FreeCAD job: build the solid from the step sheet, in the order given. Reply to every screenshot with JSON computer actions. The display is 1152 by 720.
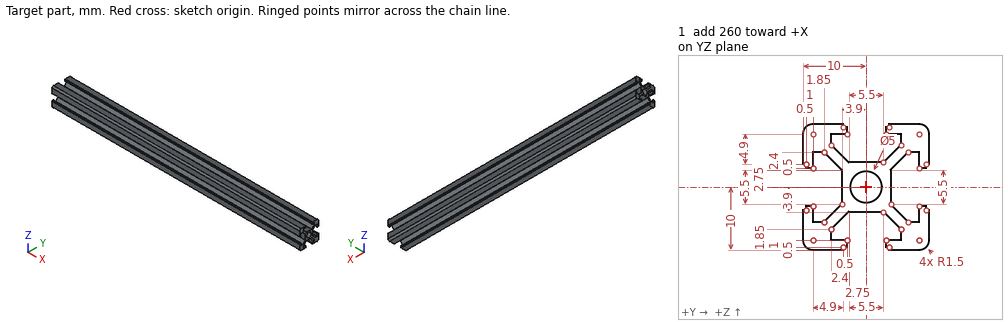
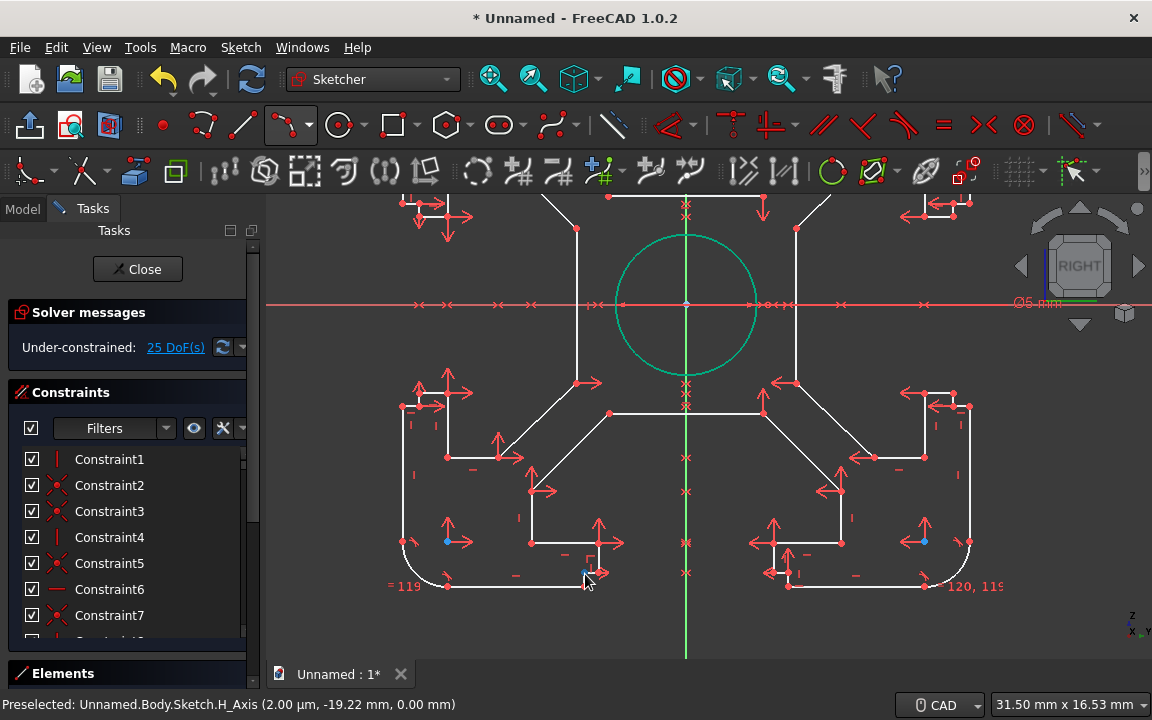
{"action": "left_click", "coordinate": [584, 573]}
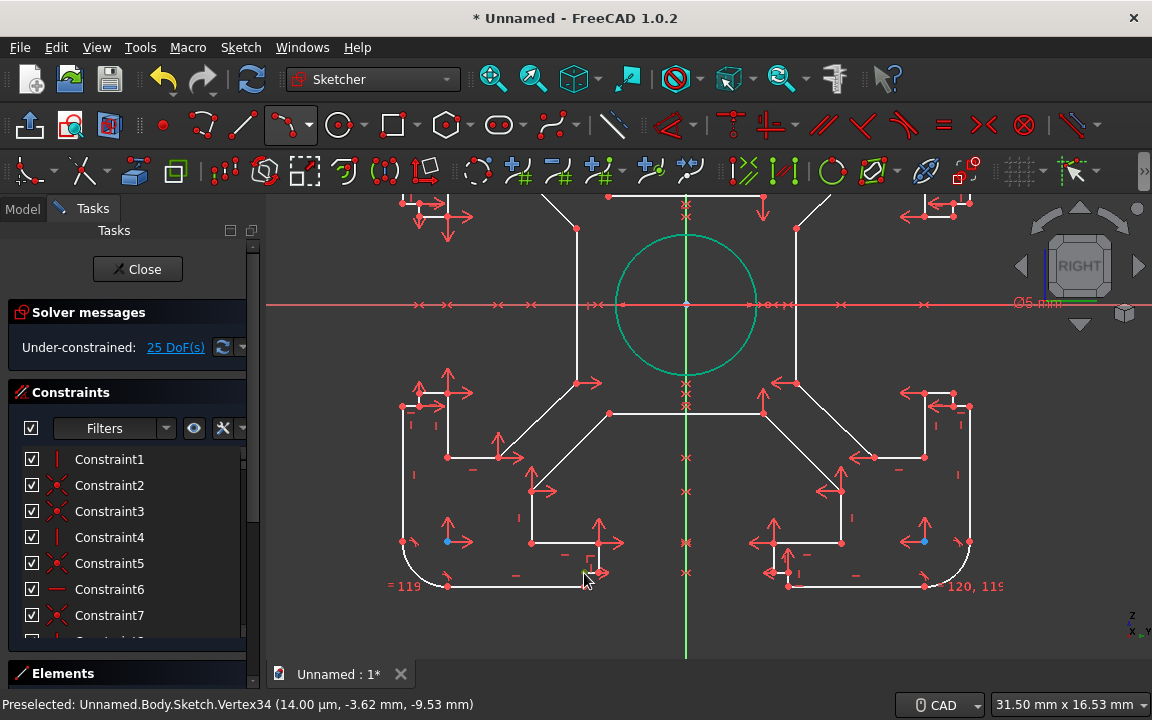
{"action": "scroll", "coordinate": [585, 574], "scroll_direction": "down", "scroll_amount": 3}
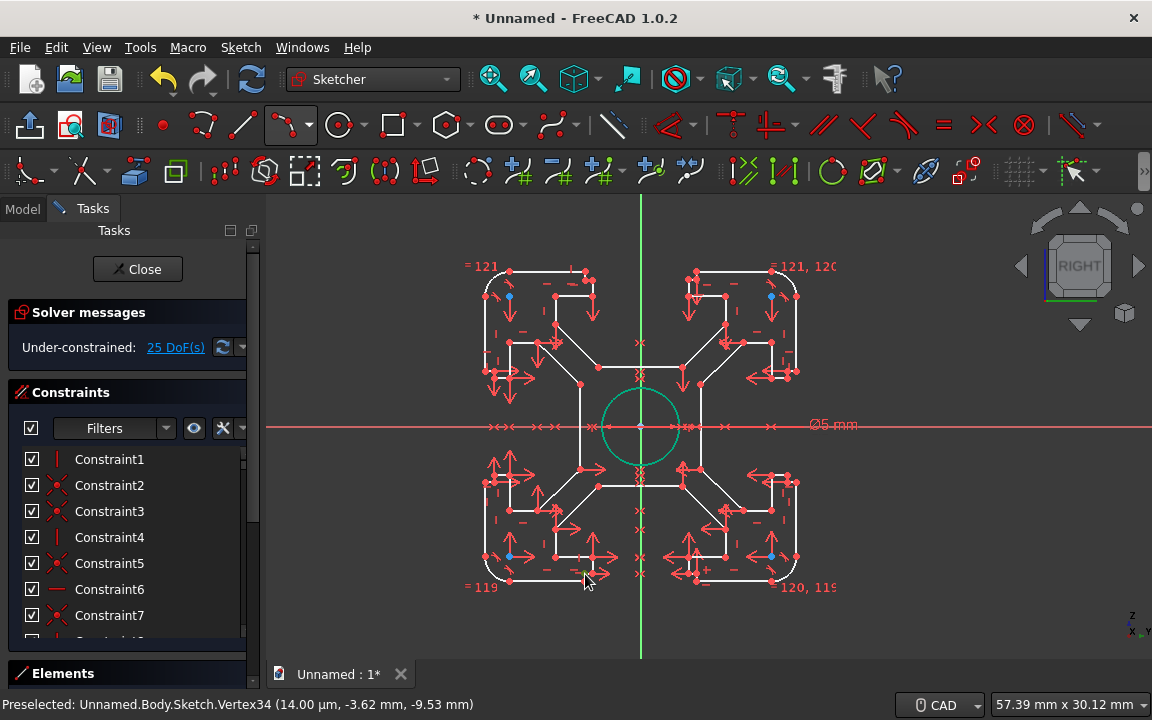
{"action": "scroll", "coordinate": [585, 280], "scroll_direction": "up", "scroll_amount": 3}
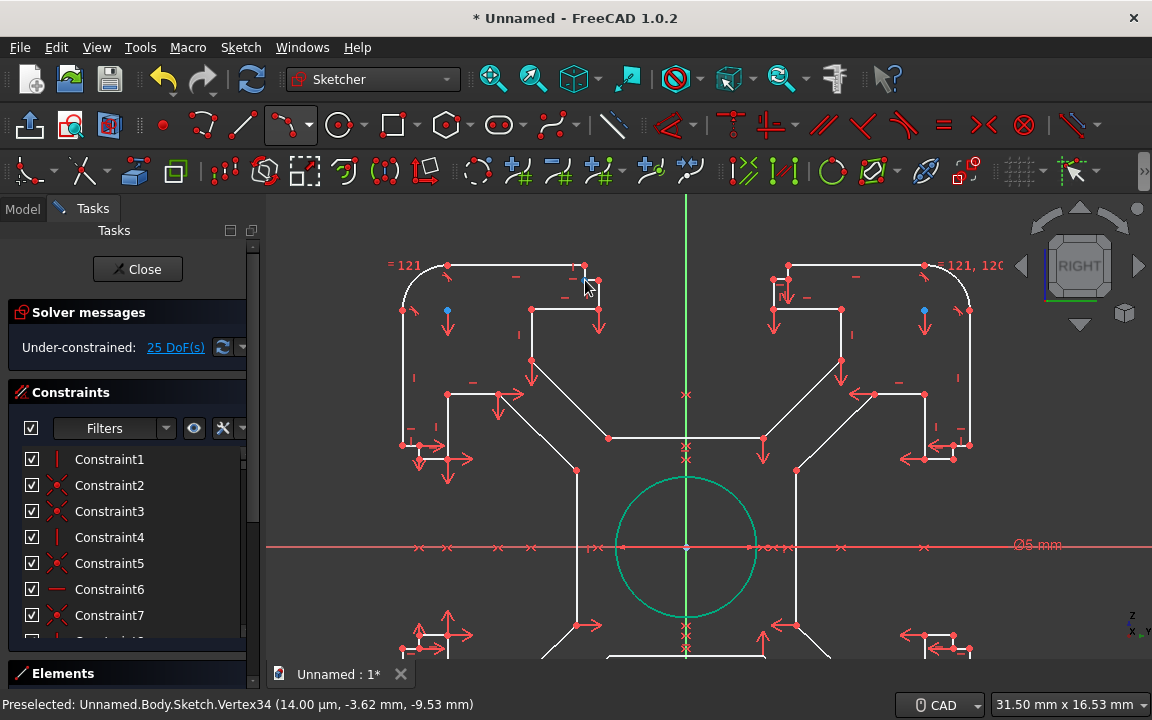
{"action": "left_click", "coordinate": [585, 280]}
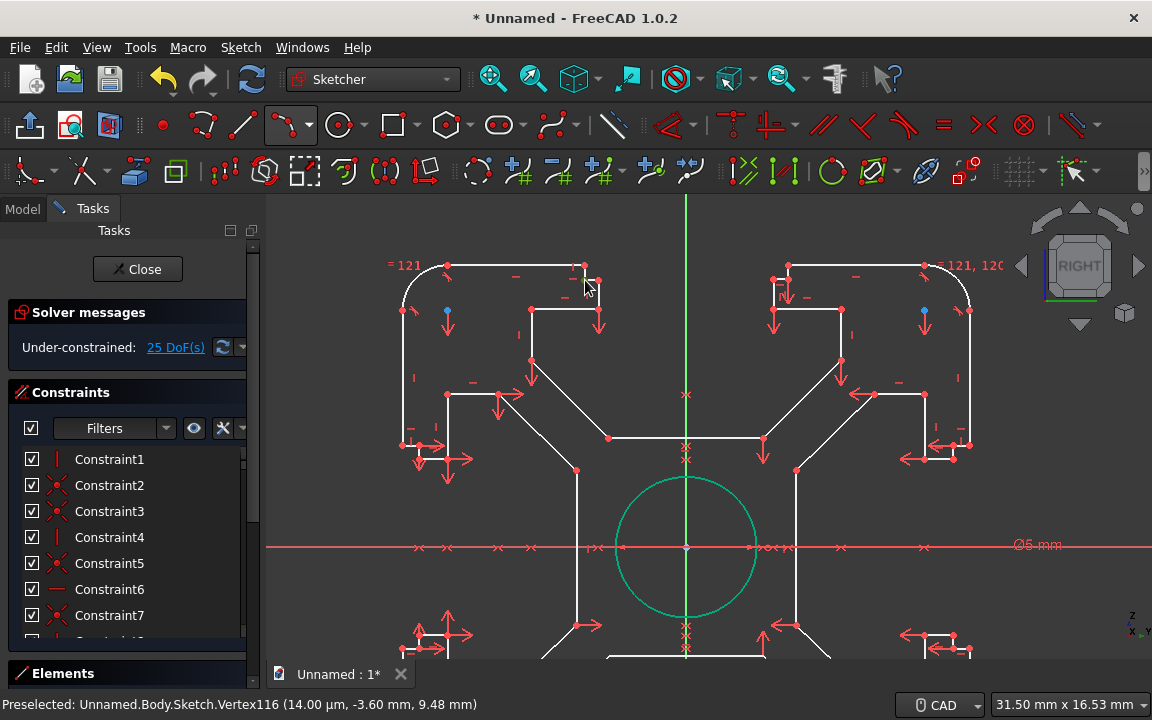
{"action": "left_click", "coordinate": [344, 547]}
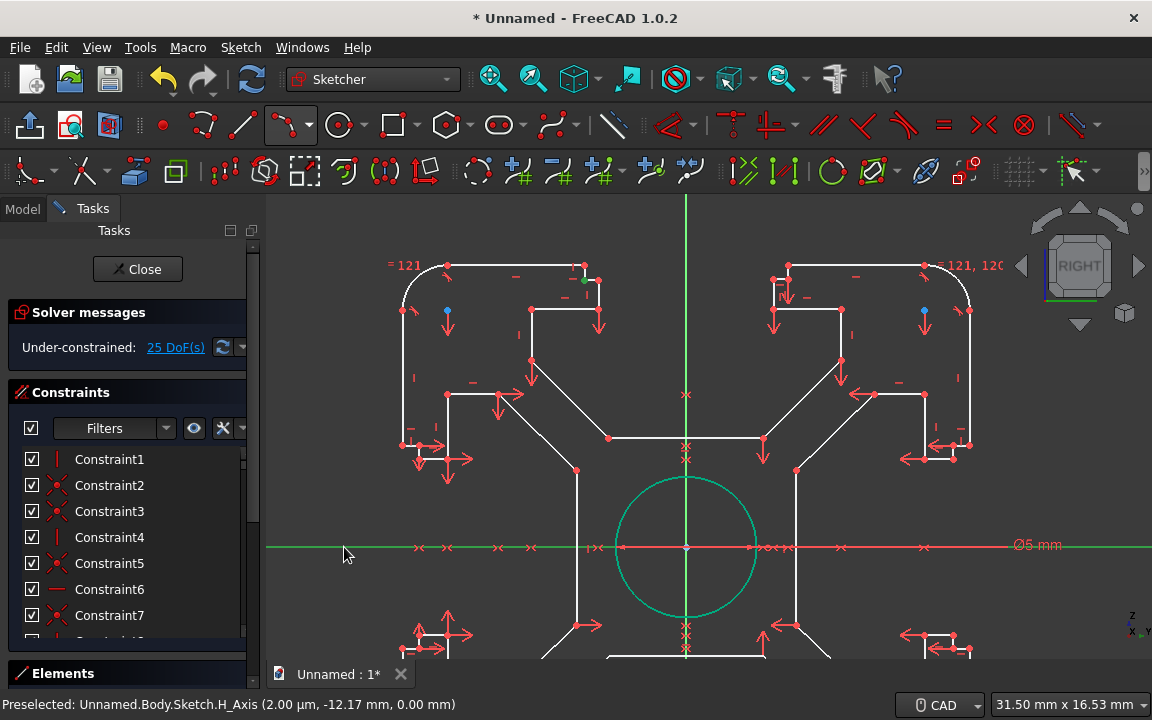
{"action": "key", "text": "s"}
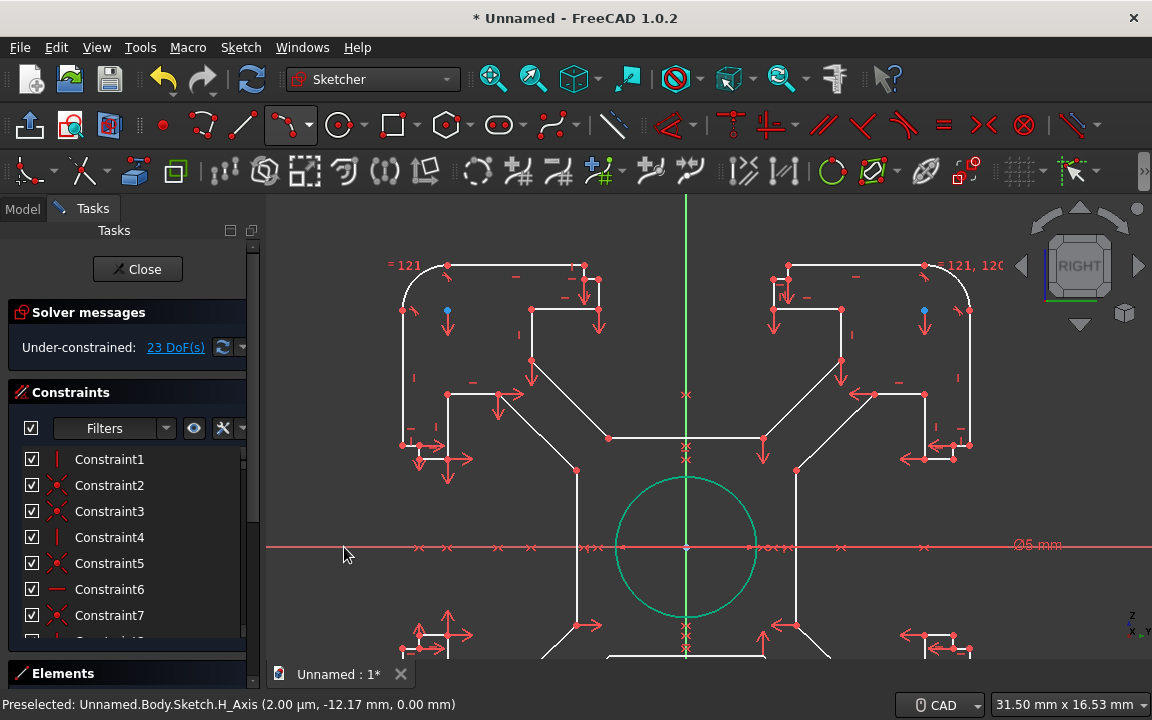
{"action": "key", "text": "d"}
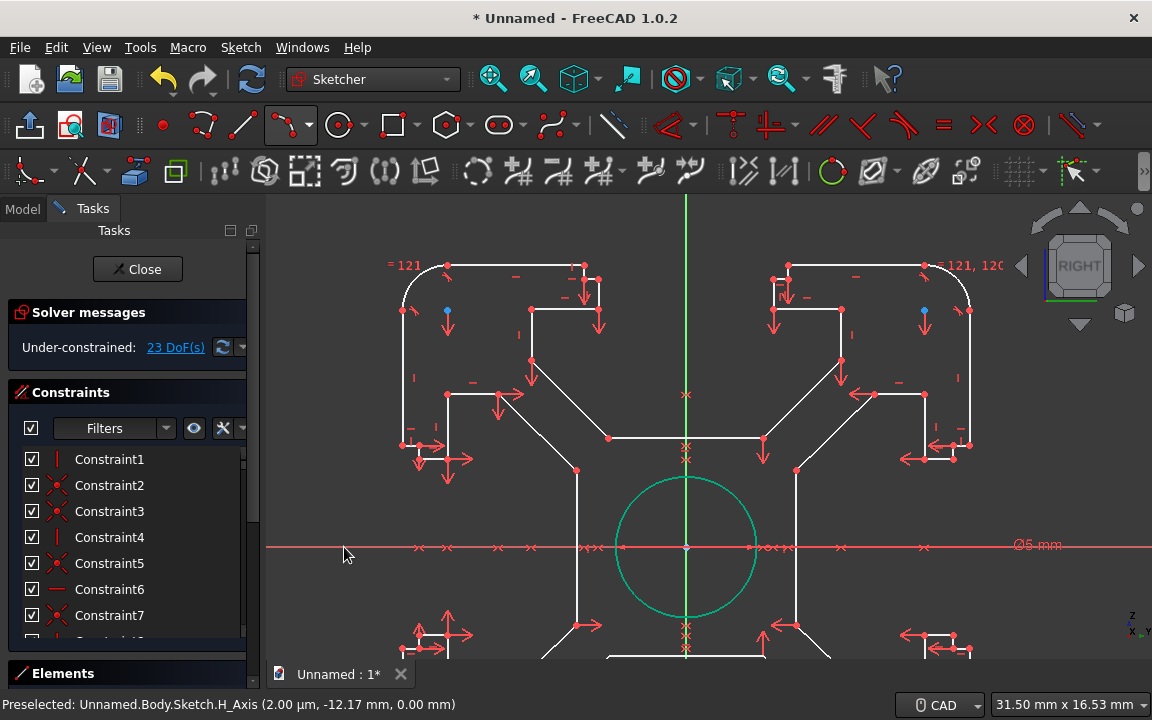
{"action": "scroll", "coordinate": [585, 280], "scroll_direction": "down", "scroll_amount": 3}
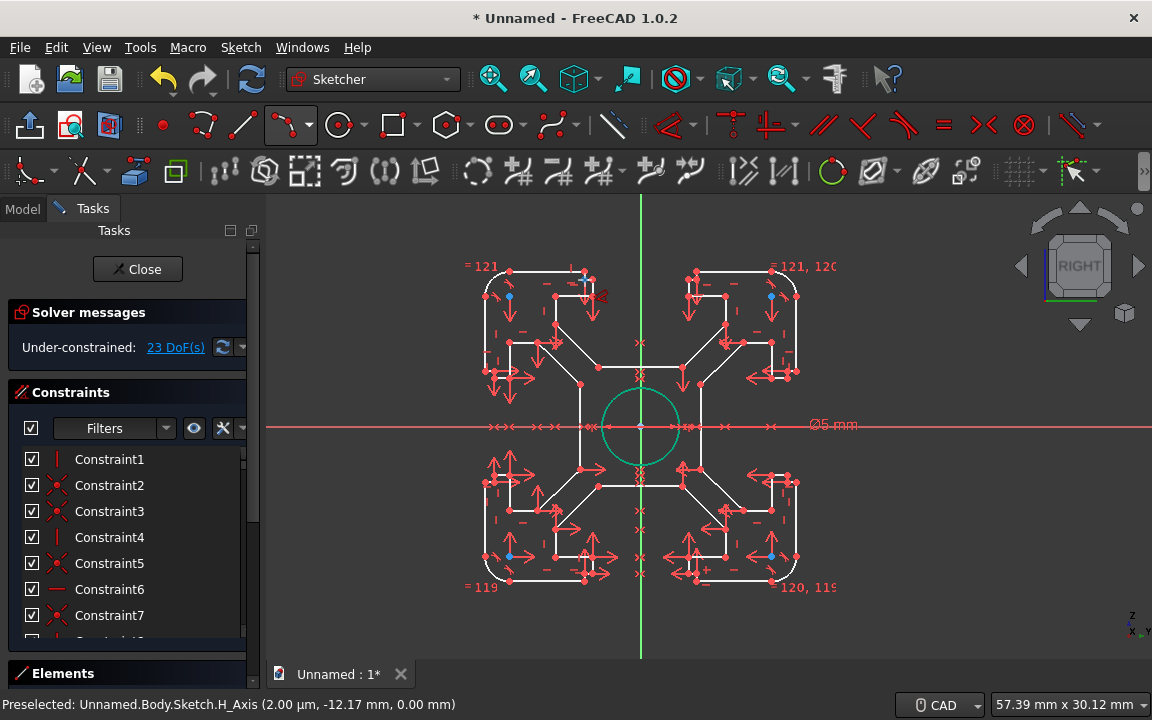
{"action": "scroll", "coordinate": [488, 568], "scroll_direction": "up", "scroll_amount": 3}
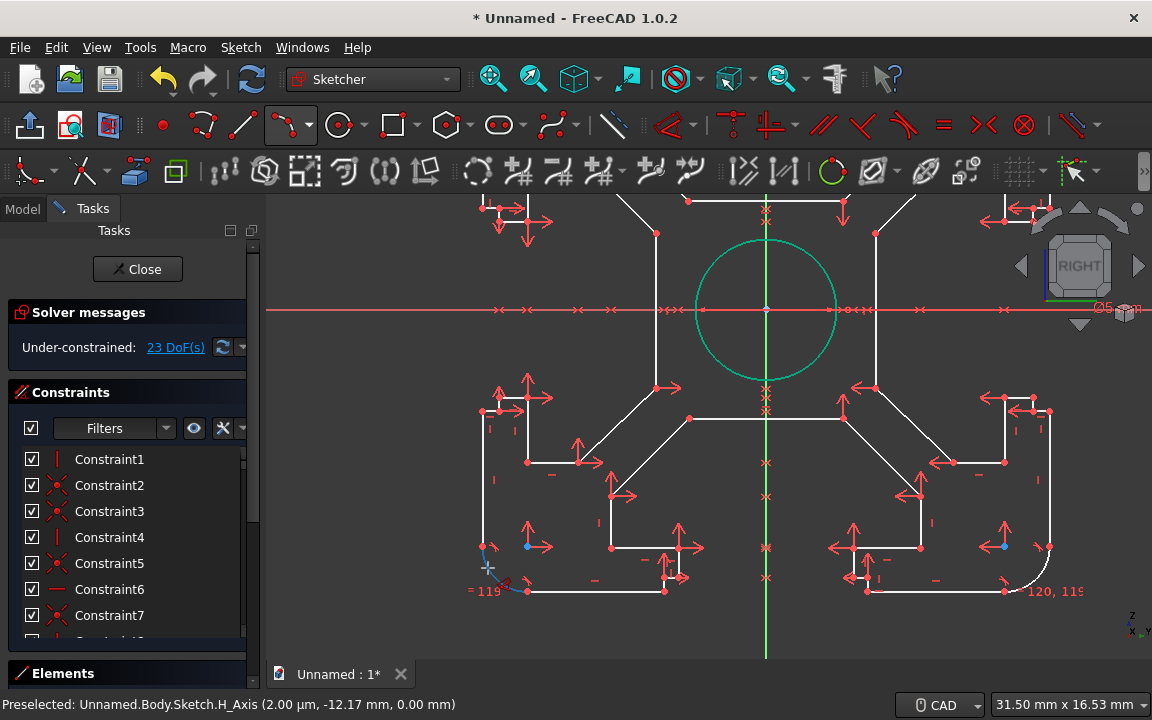
{"action": "left_click", "coordinate": [487, 567]}
{"action": "left_click", "coordinate": [458, 581]}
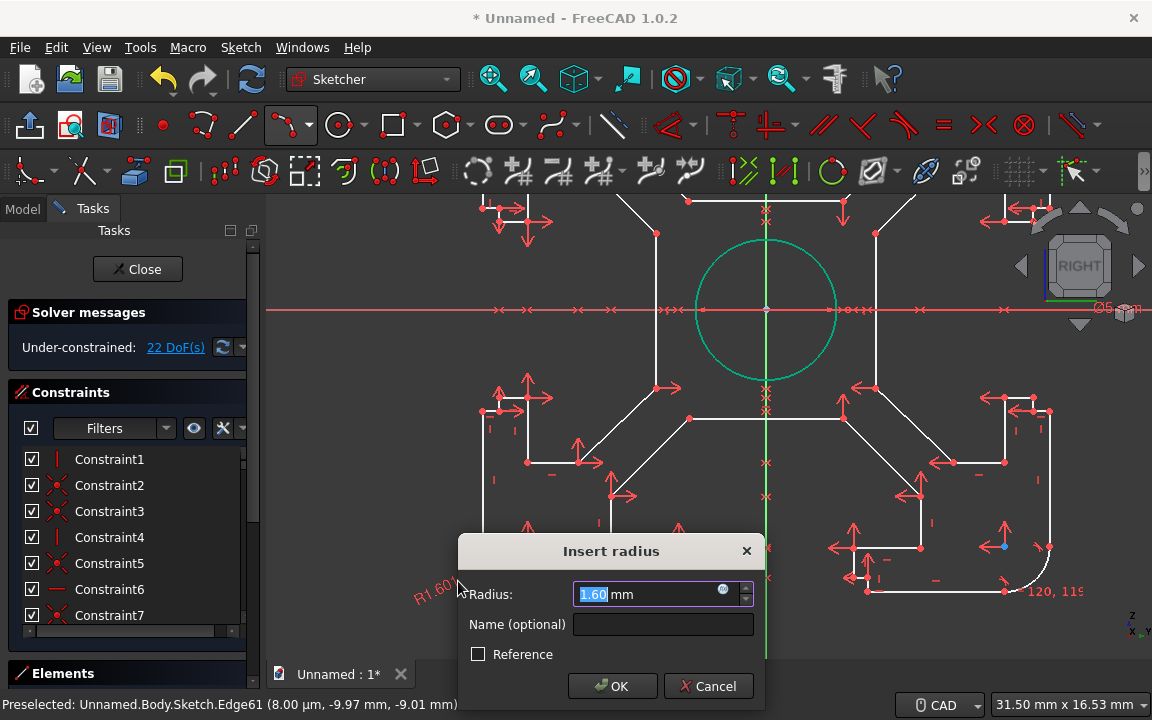
{"action": "type", "text": "1.5"}
{"action": "key", "text": "Return"}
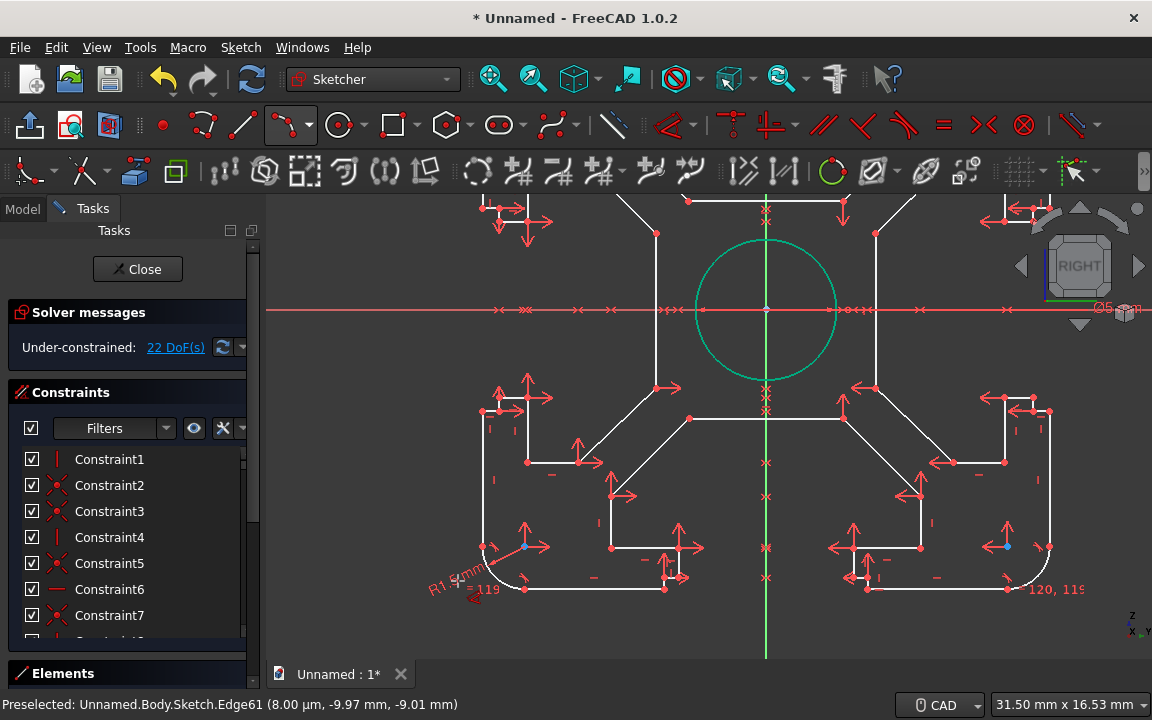
{"action": "scroll", "coordinate": [488, 568], "scroll_direction": "down", "scroll_amount": 3}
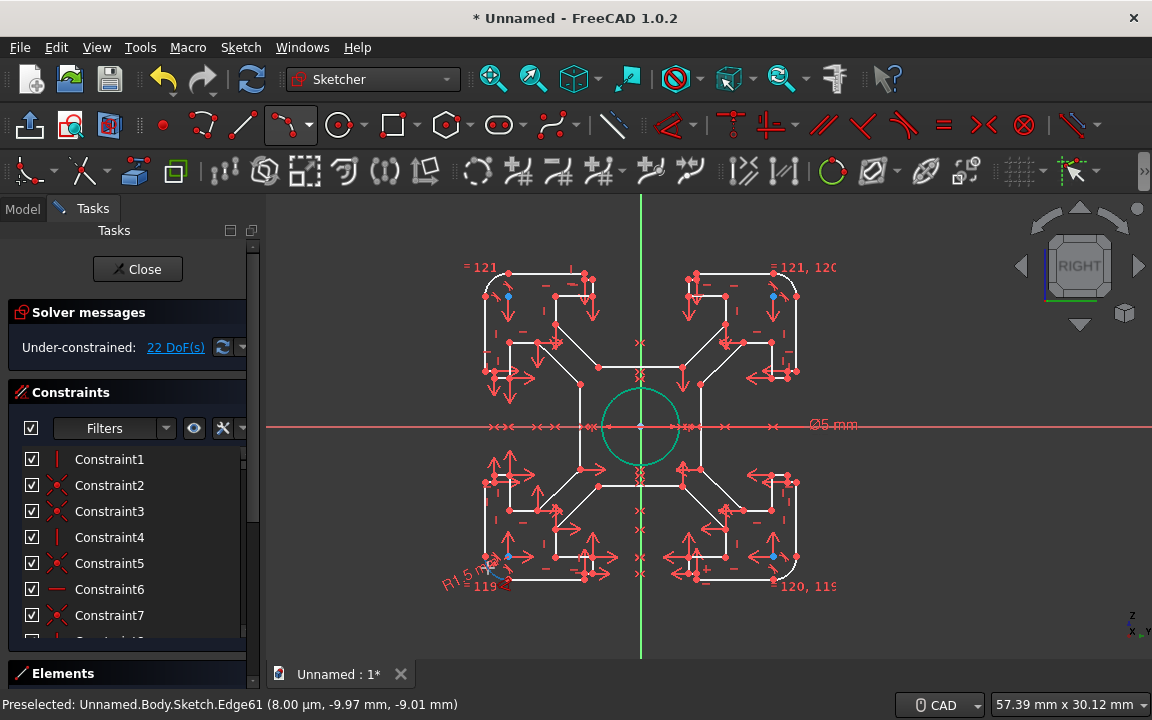
{"action": "scroll", "coordinate": [500, 378], "scroll_direction": "up", "scroll_amount": 5}